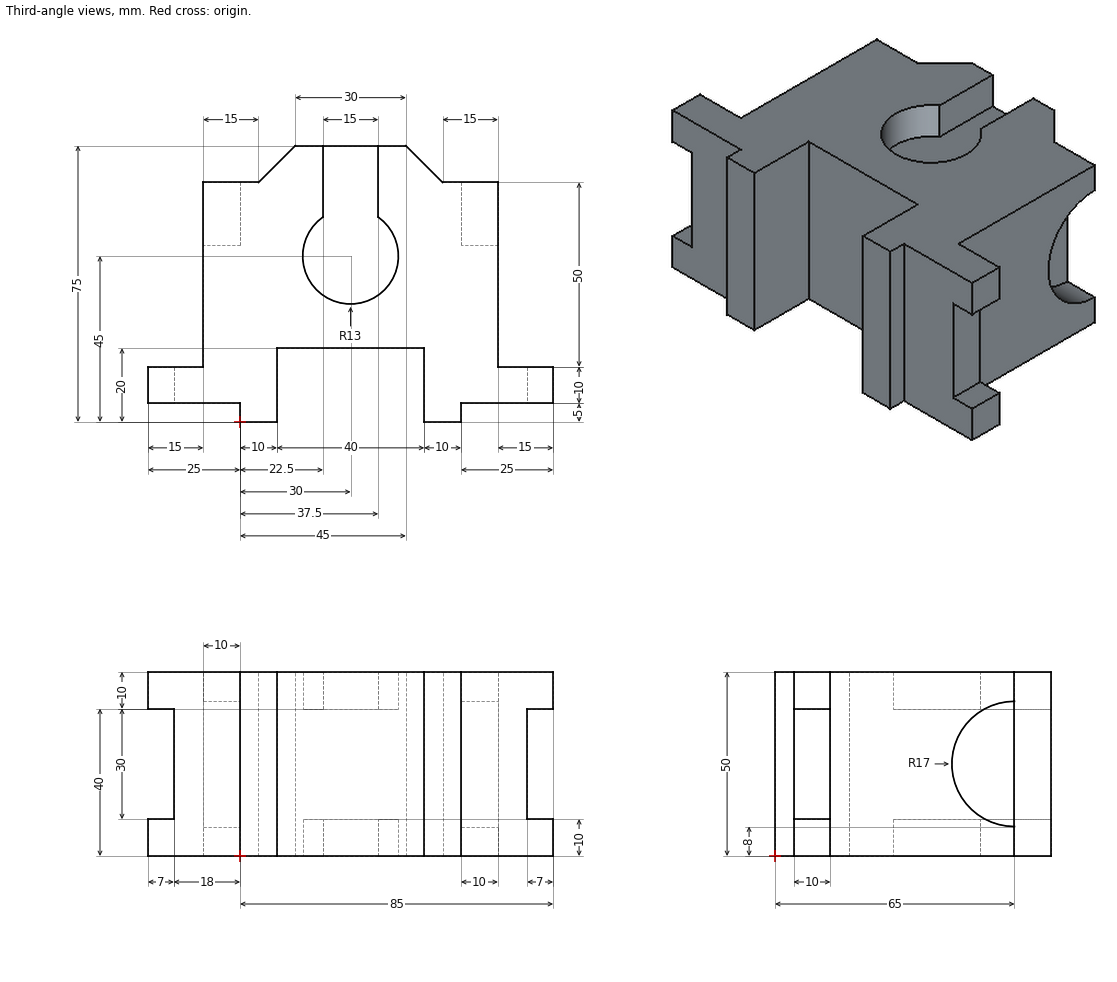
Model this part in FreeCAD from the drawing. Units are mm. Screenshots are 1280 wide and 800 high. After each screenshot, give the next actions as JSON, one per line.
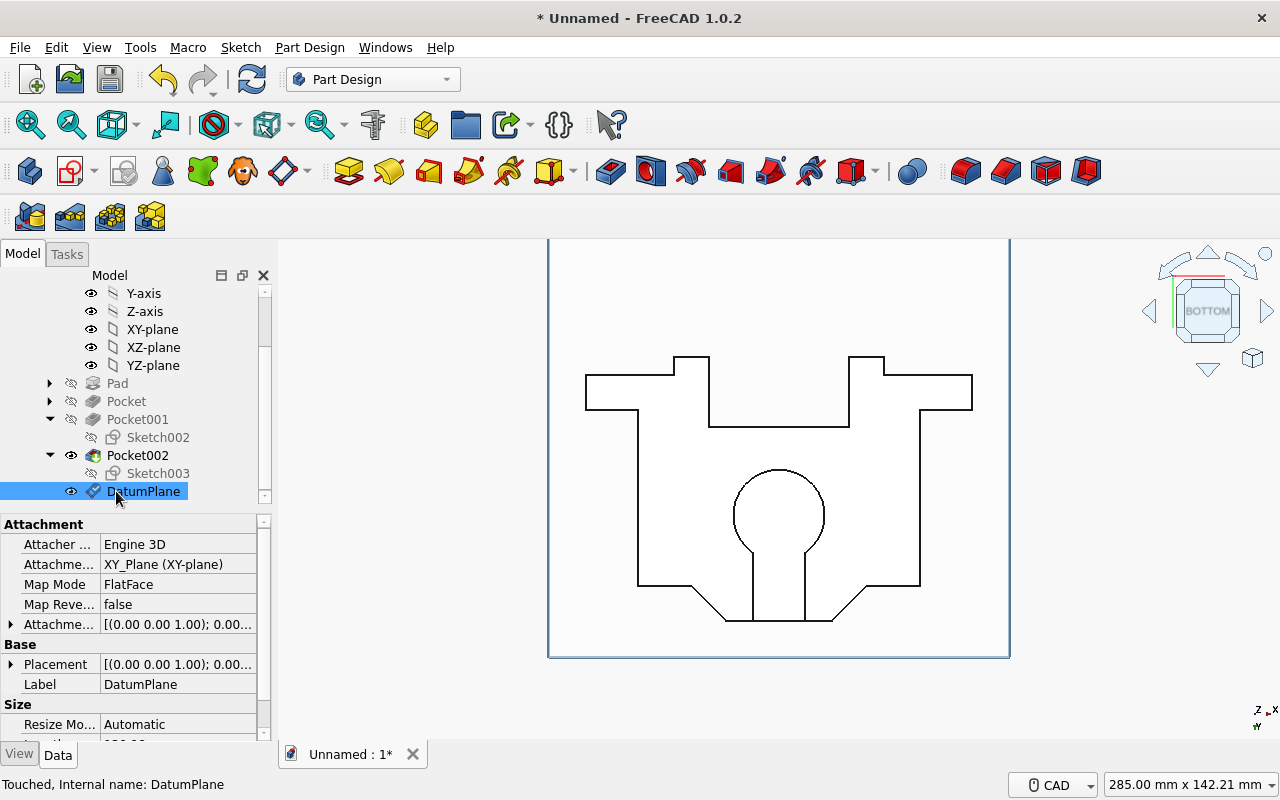
{"action": "left_click", "coordinate": [70, 172]}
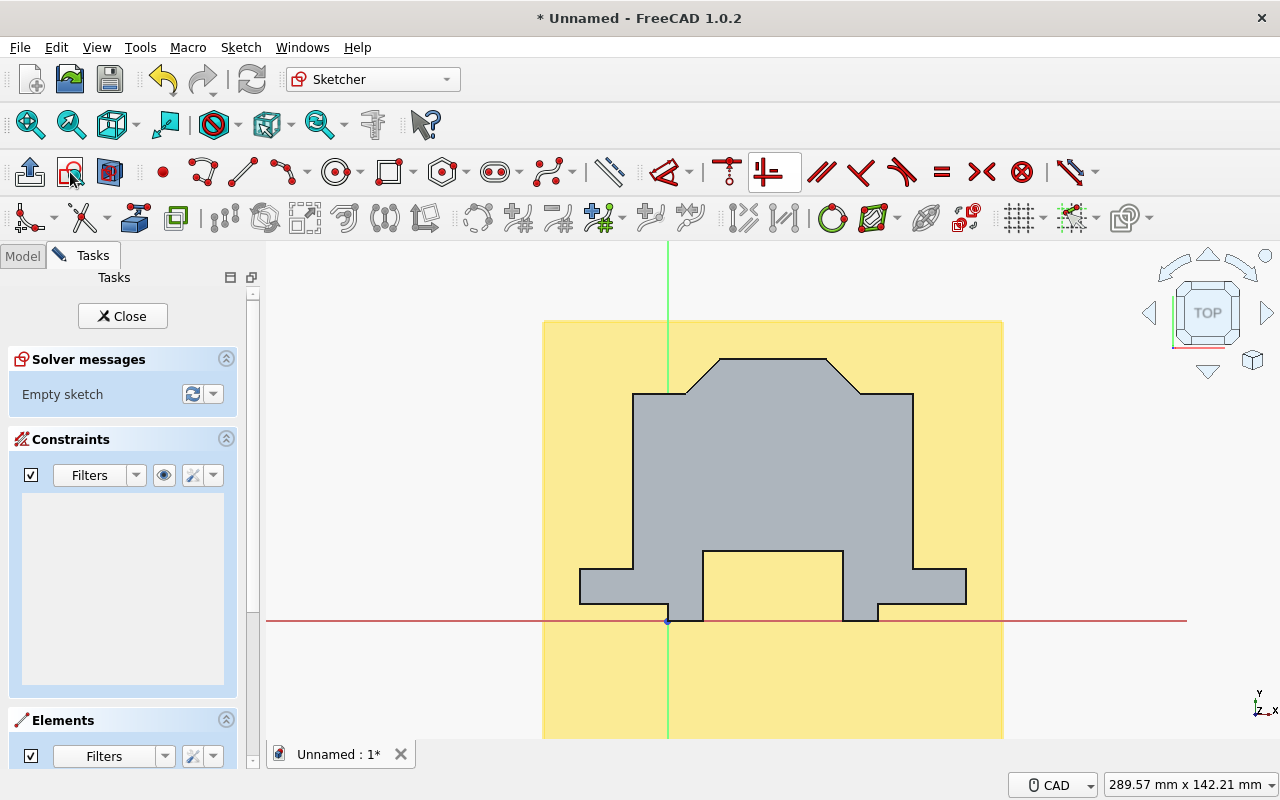
{"action": "left_click", "coordinate": [110, 172]}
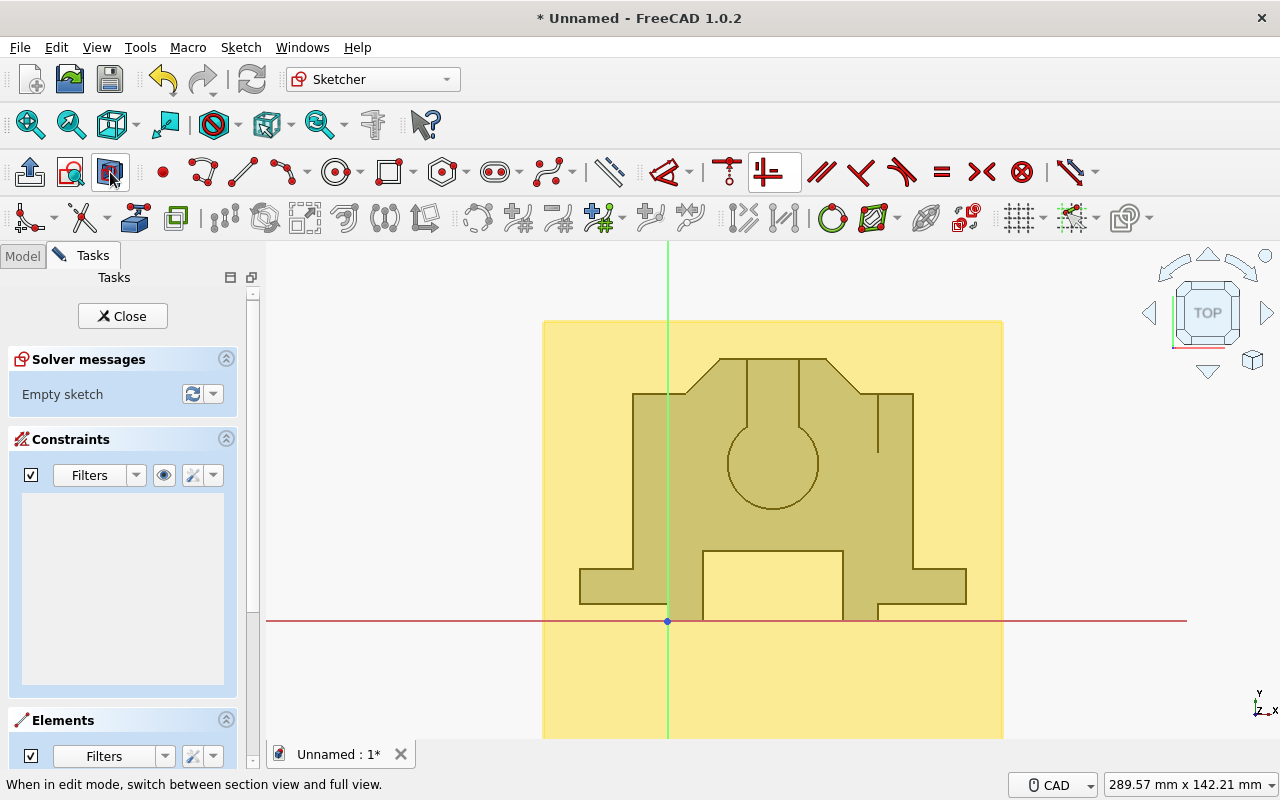
{"action": "left_click", "coordinate": [204, 172]}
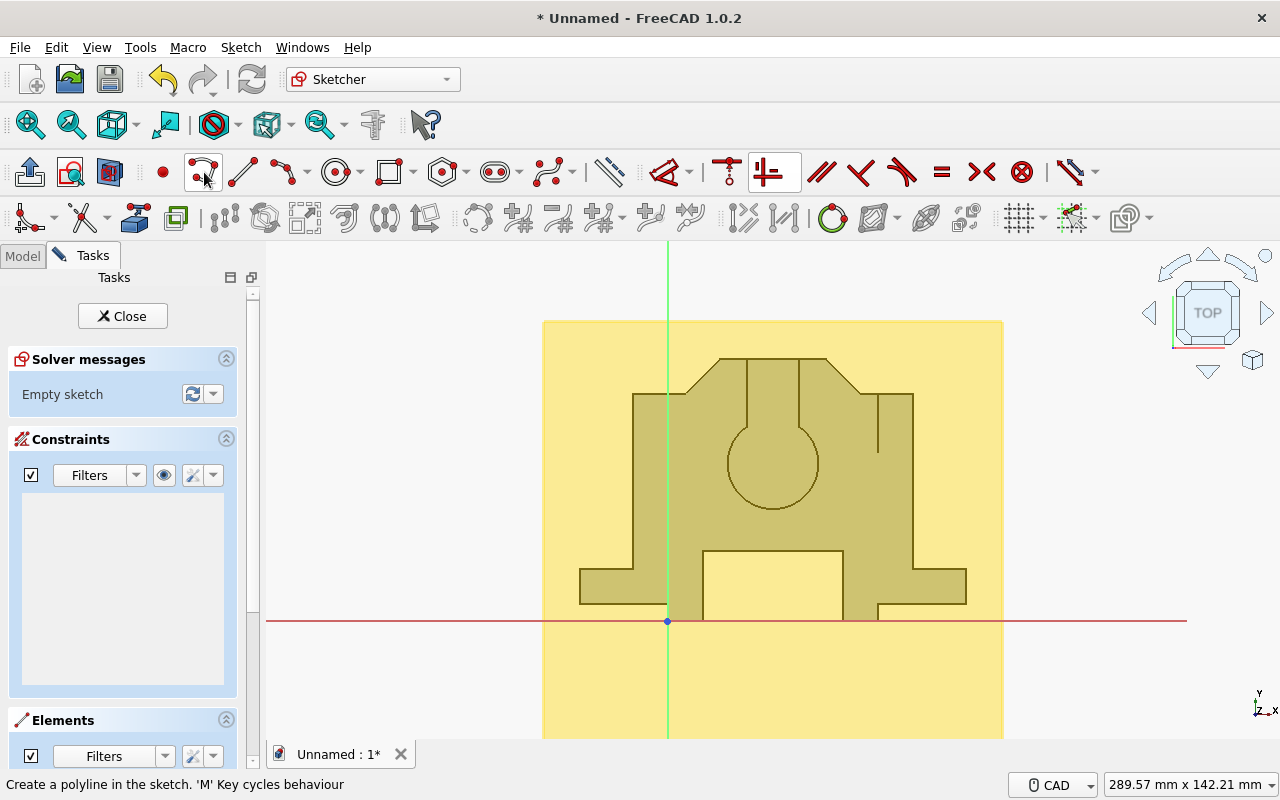
{"action": "left_click", "coordinate": [799, 427]}
{"action": "left_click", "coordinate": [799, 359]}
{"action": "left_click", "coordinate": [747, 359]}
{"action": "left_click", "coordinate": [747, 427]}
{"action": "right_click", "coordinate": [747, 427]}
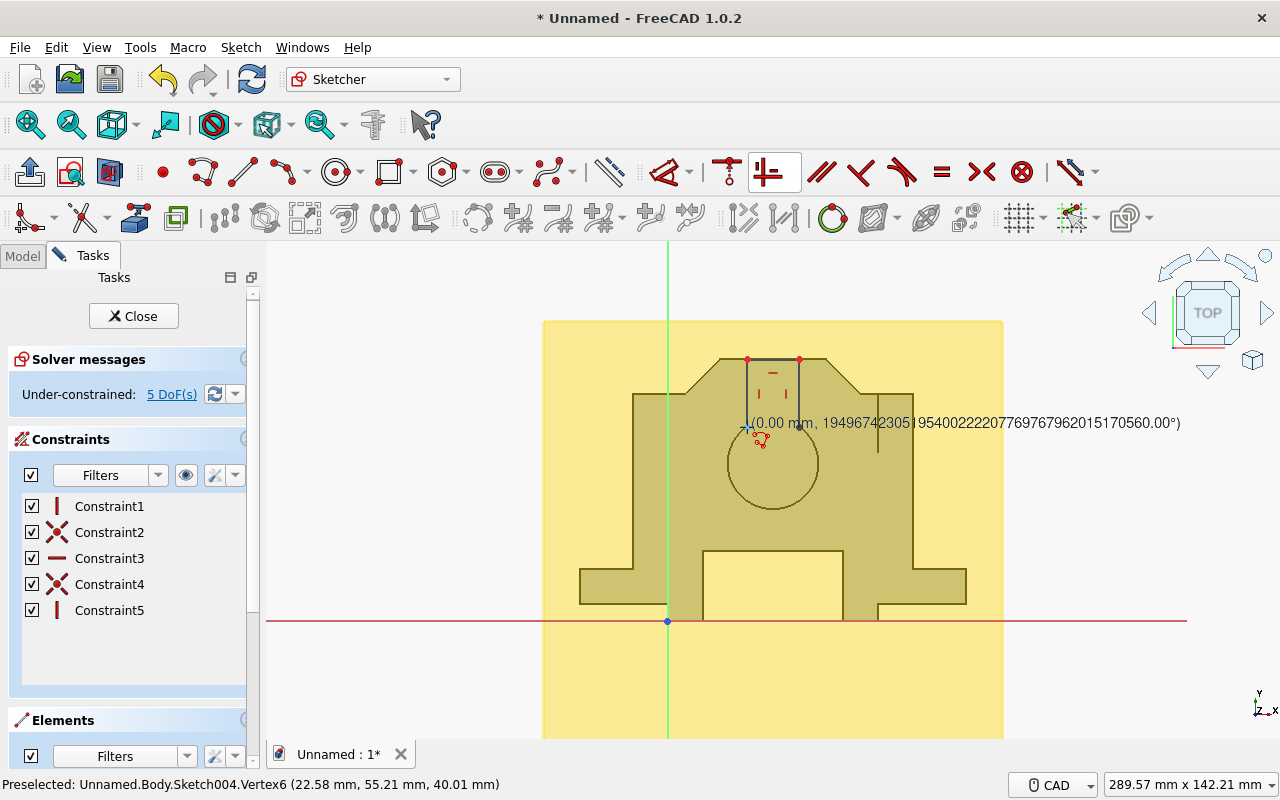
{"action": "left_click", "coordinate": [284, 172]}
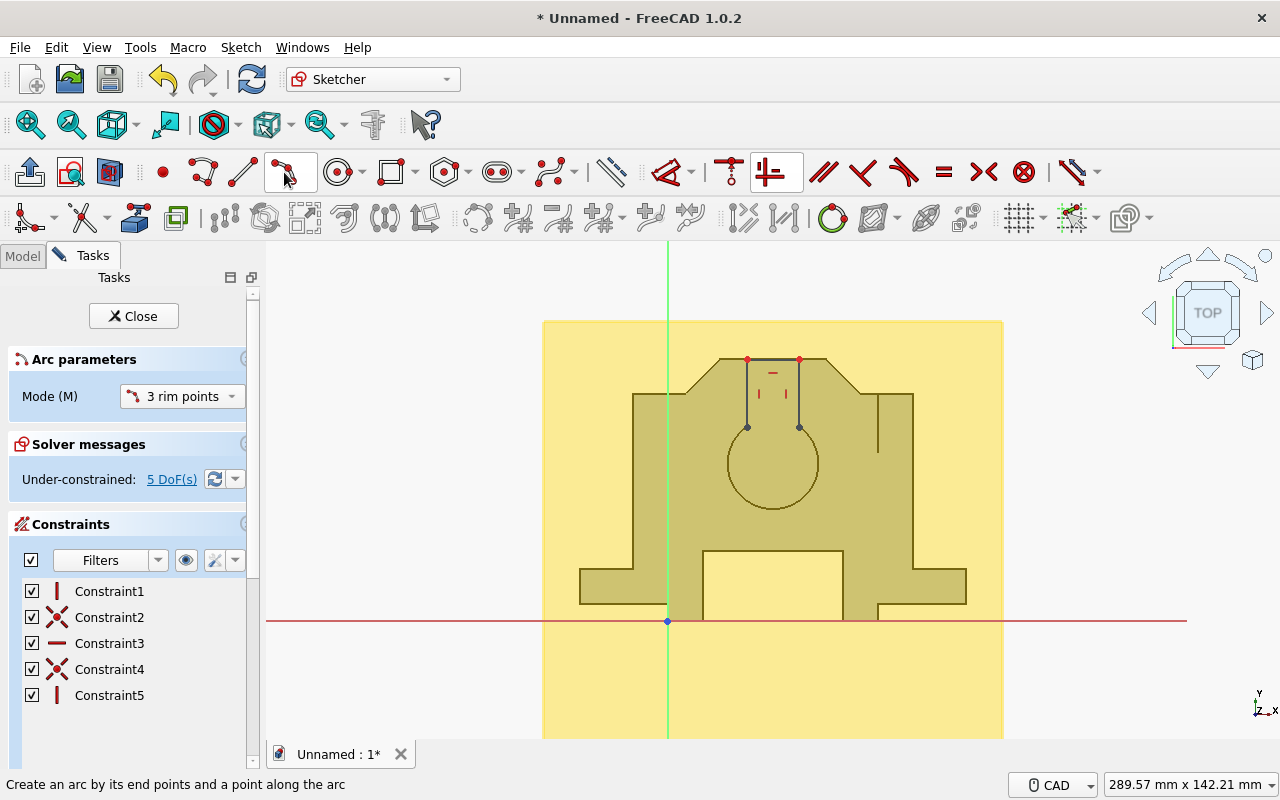
{"action": "left_click", "coordinate": [747, 428]}
{"action": "left_click", "coordinate": [799, 428]}
{"action": "left_click", "coordinate": [773, 509]}
{"action": "key", "text": "Escape"}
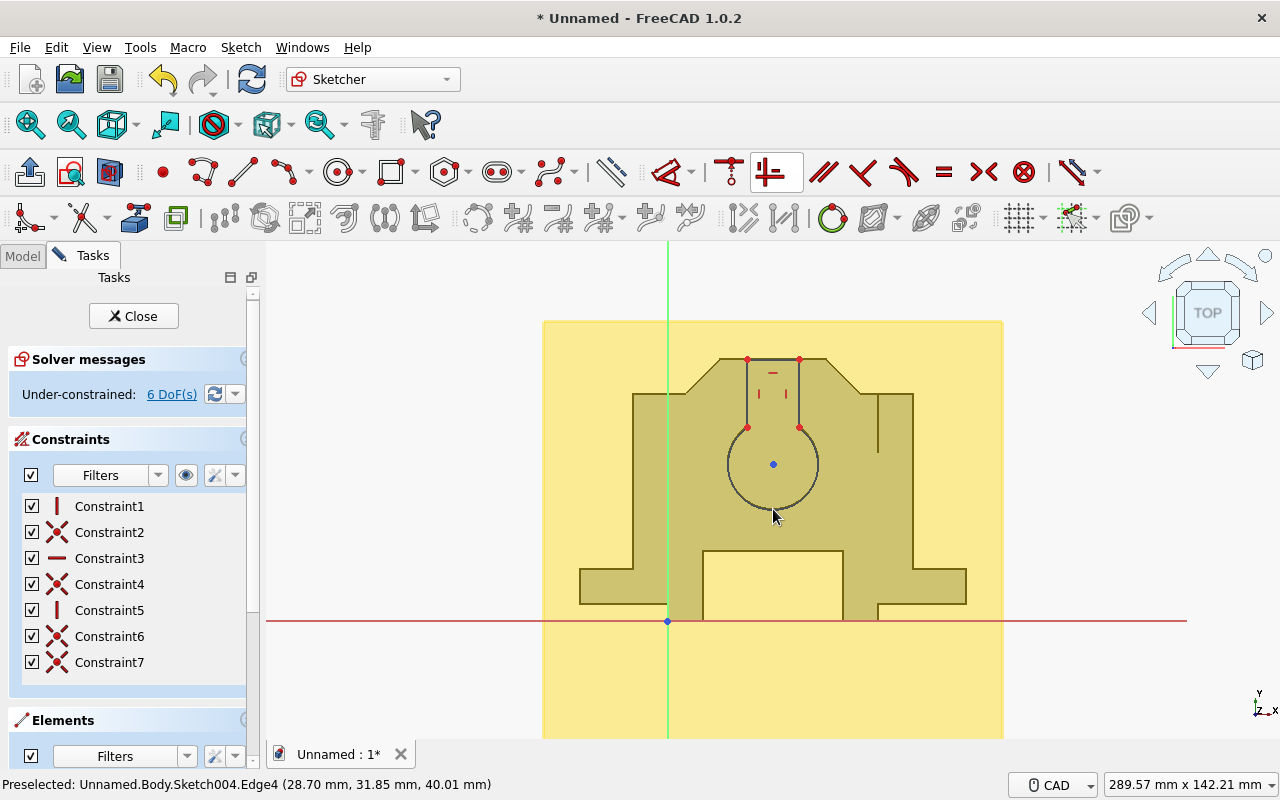
{"action": "left_click", "coordinate": [666, 172]}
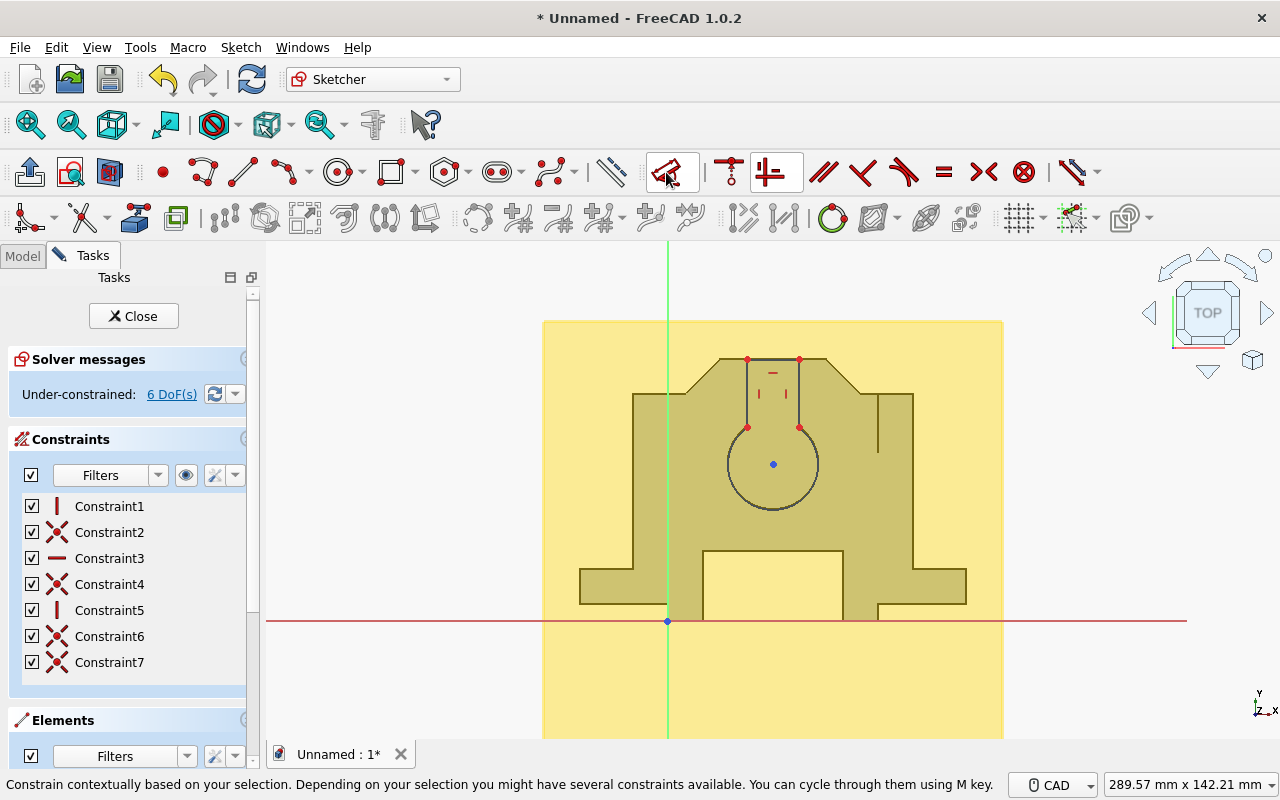
{"action": "left_click", "coordinate": [735, 489]}
{"action": "left_click", "coordinate": [708, 506]}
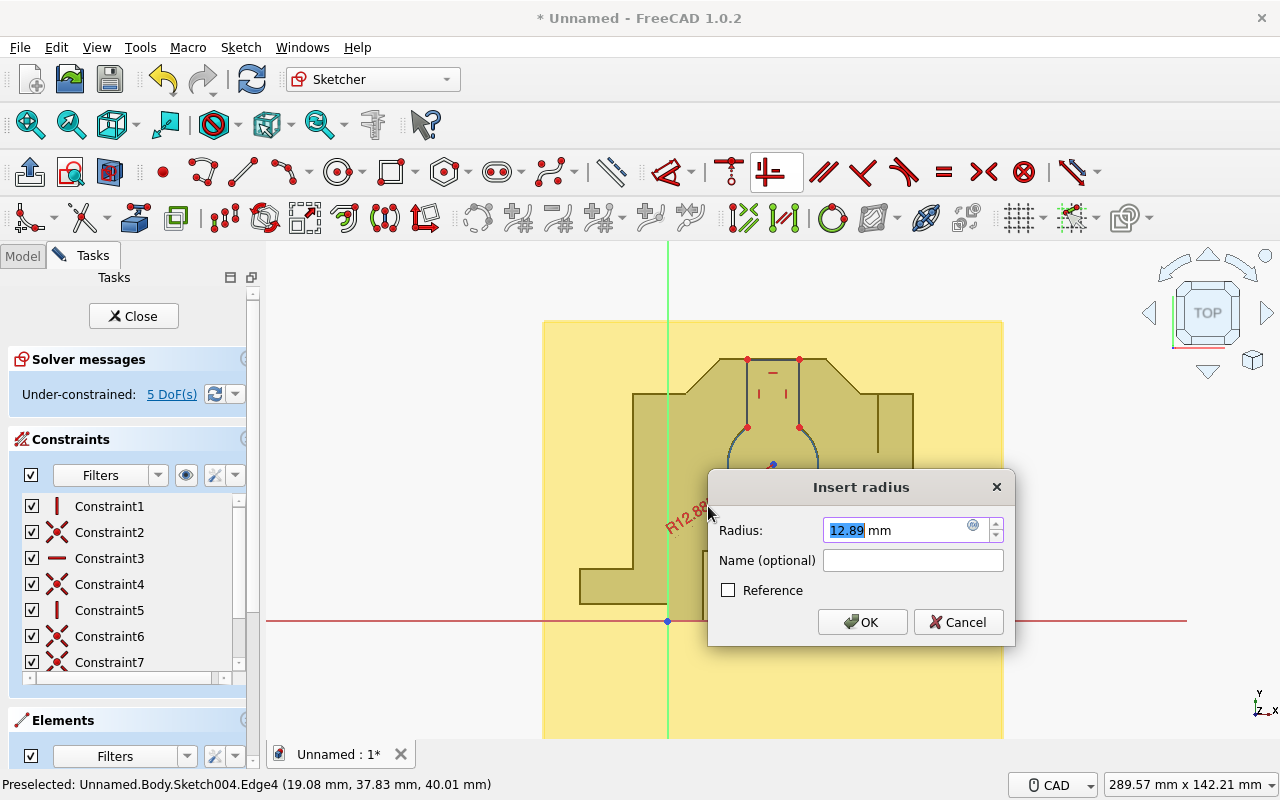
{"action": "type", "text": "13"}
{"action": "key", "text": "Return"}